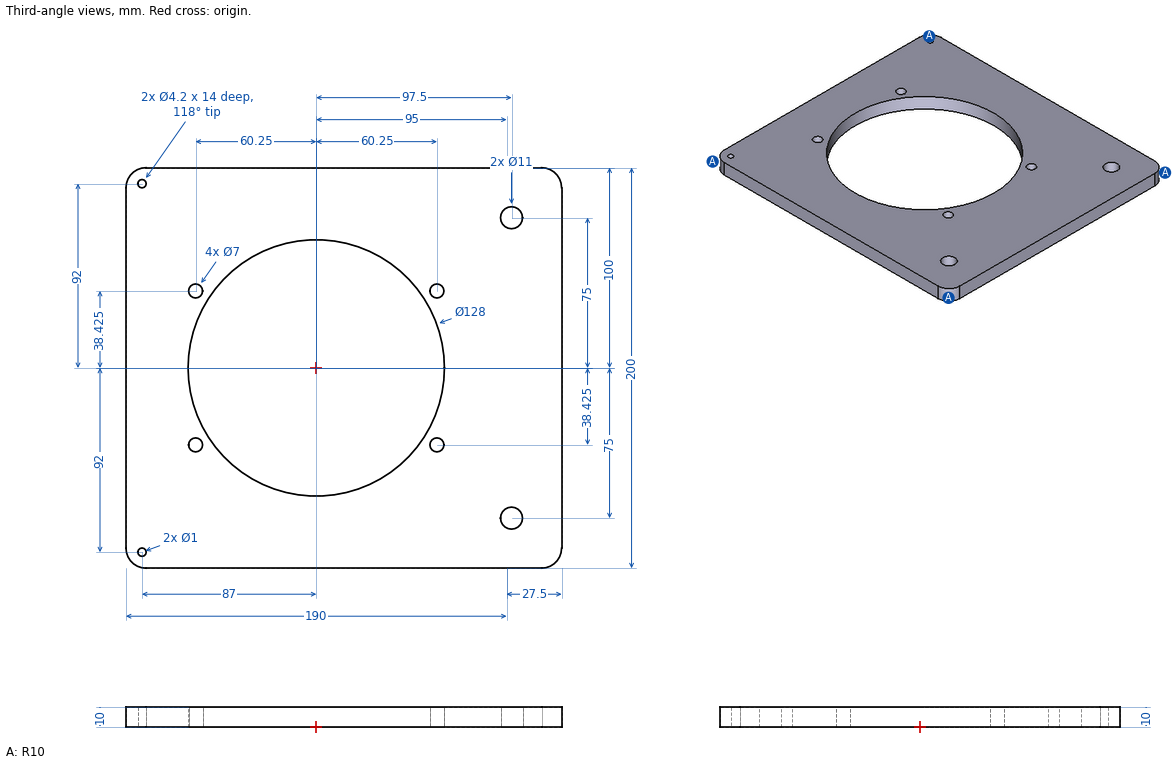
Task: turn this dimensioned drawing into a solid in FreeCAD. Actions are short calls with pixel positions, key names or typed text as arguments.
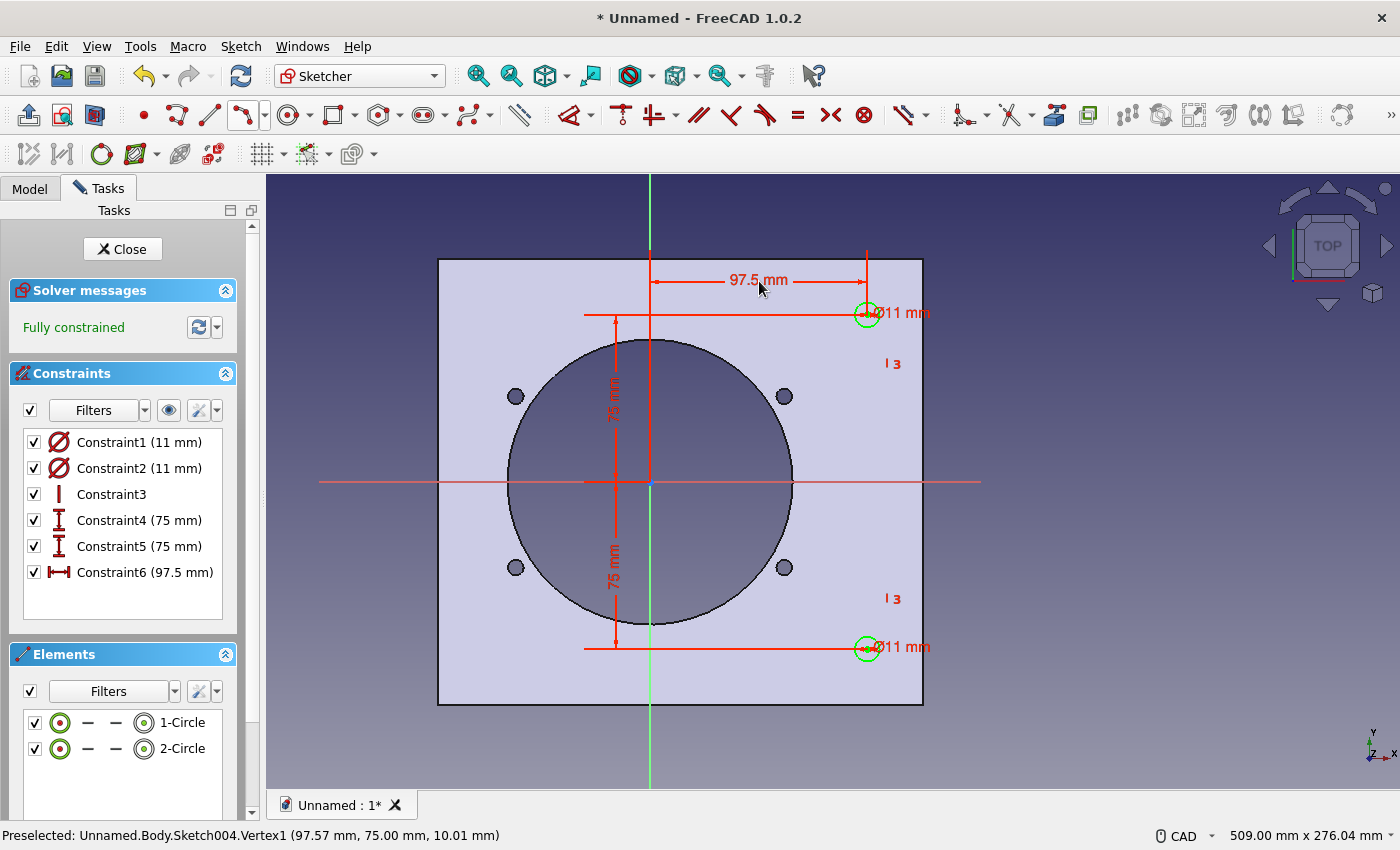
click(123, 249)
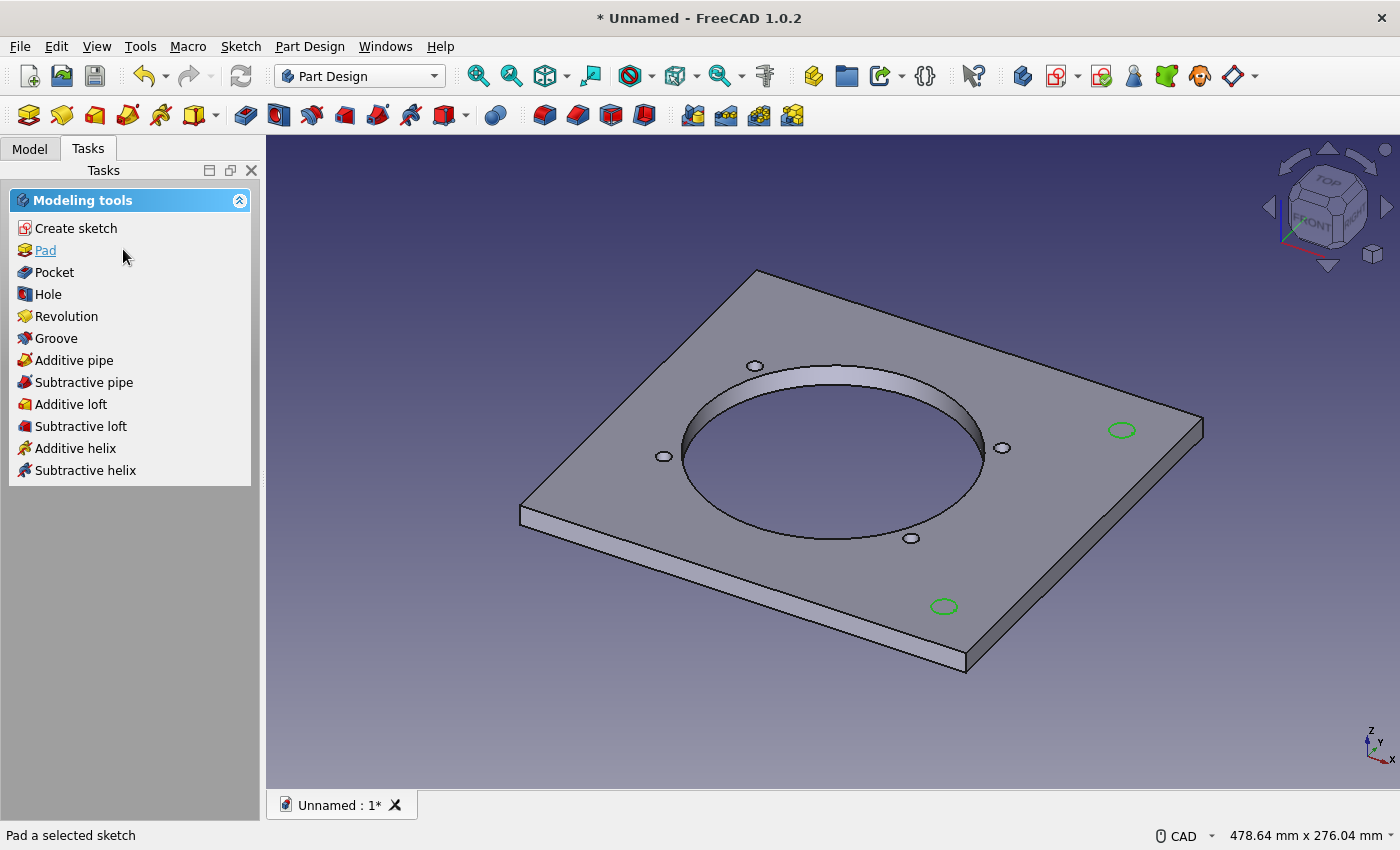
click(246, 116)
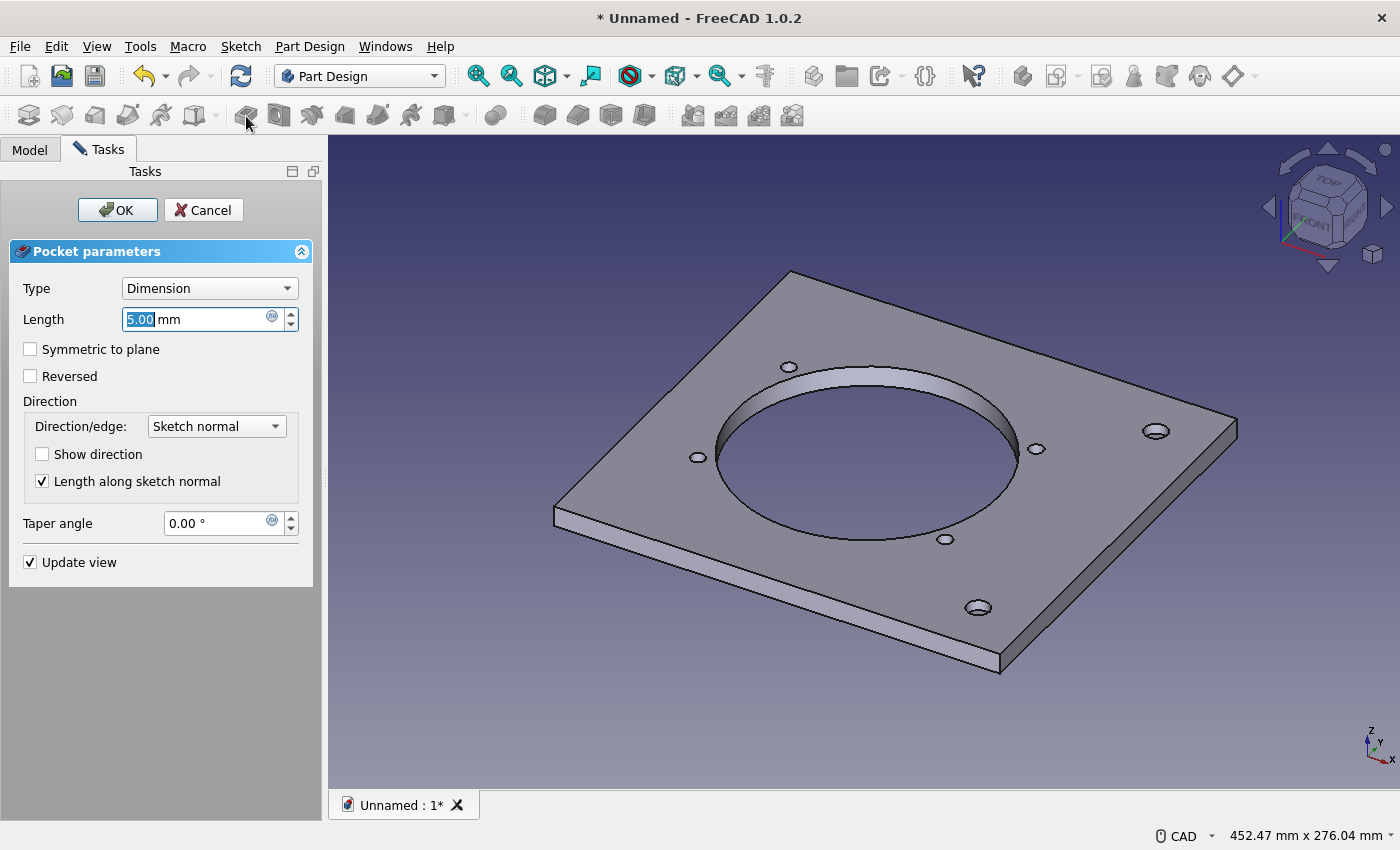
text(10)
key(Tab)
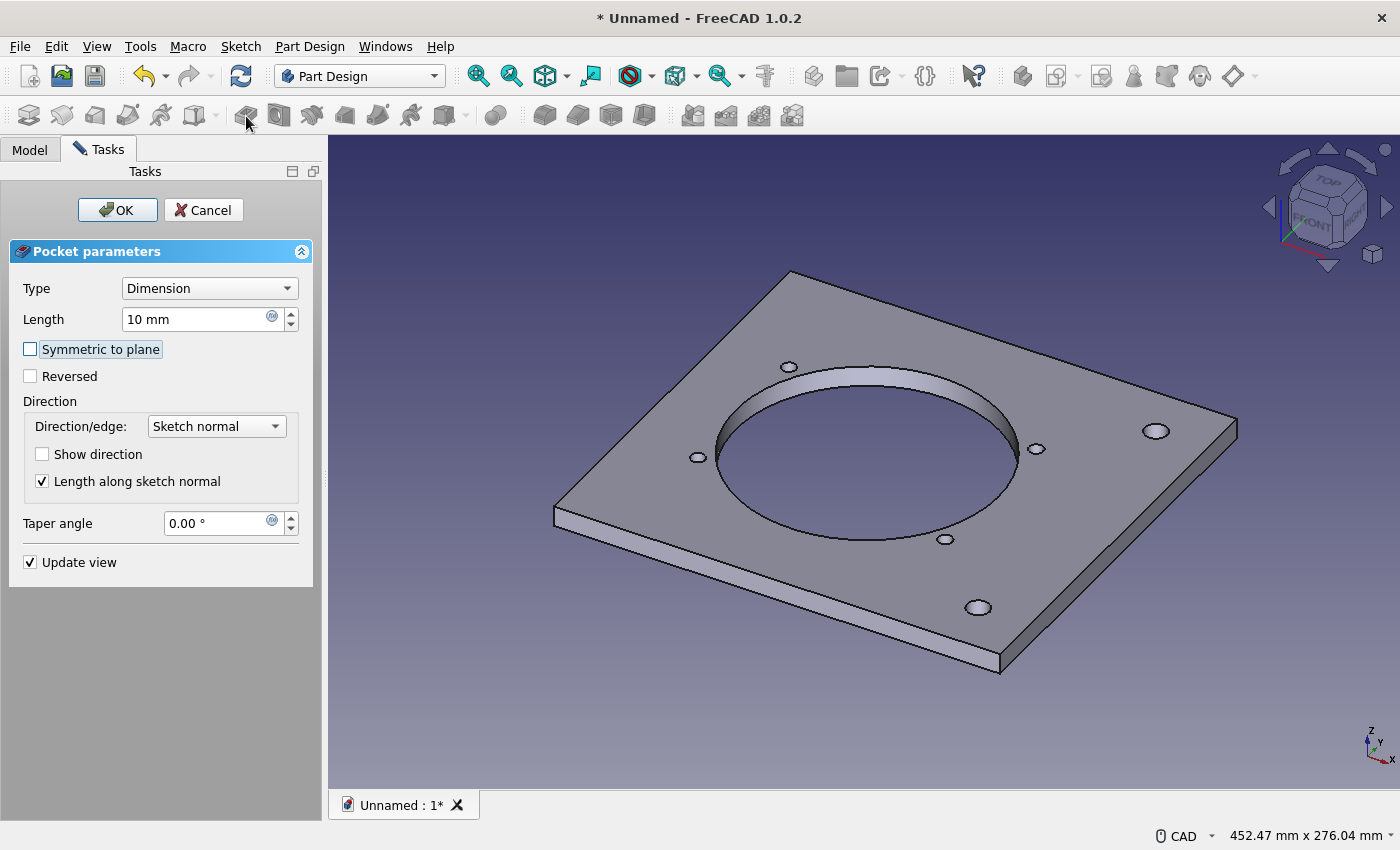
click(118, 210)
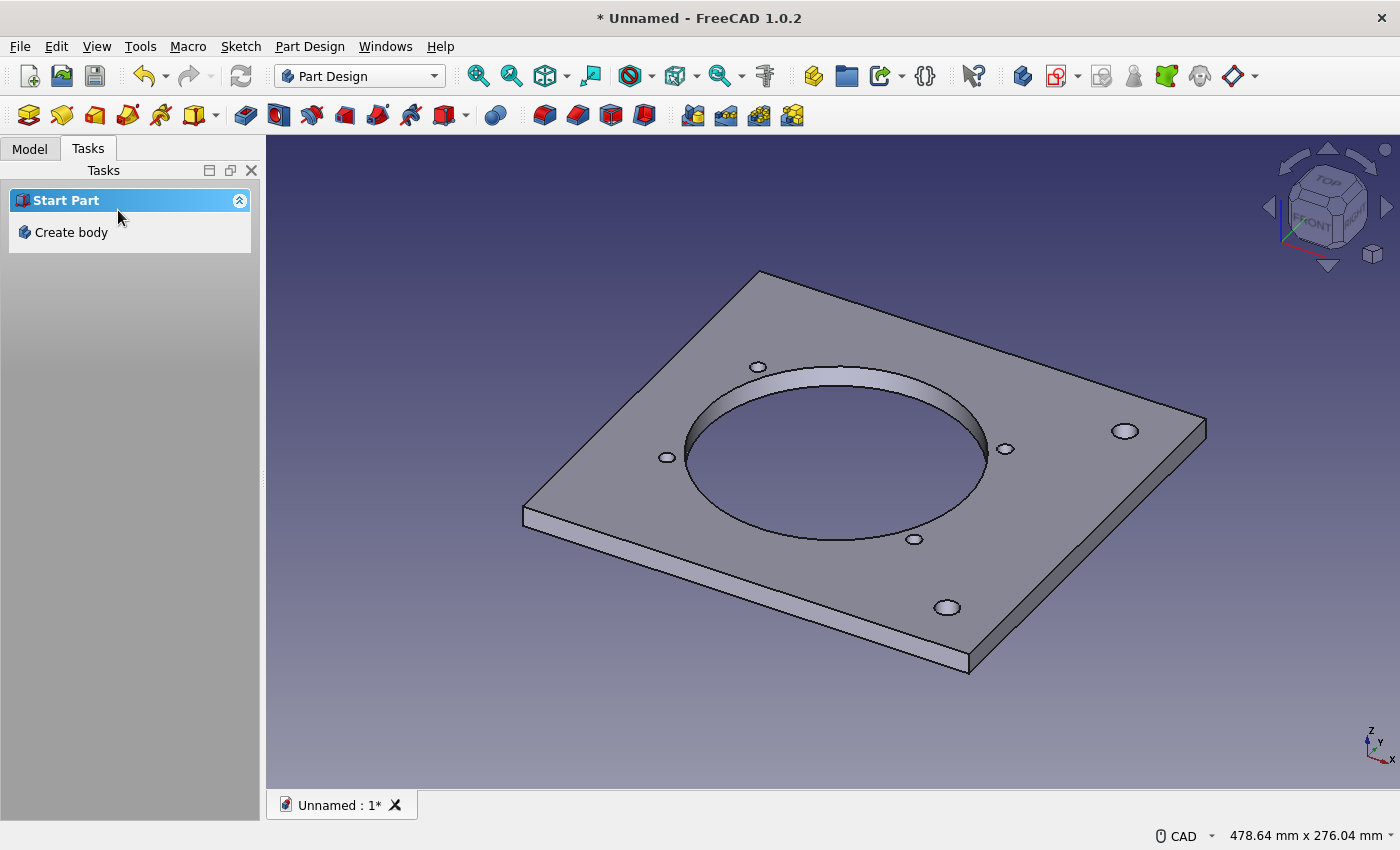
click(924, 571)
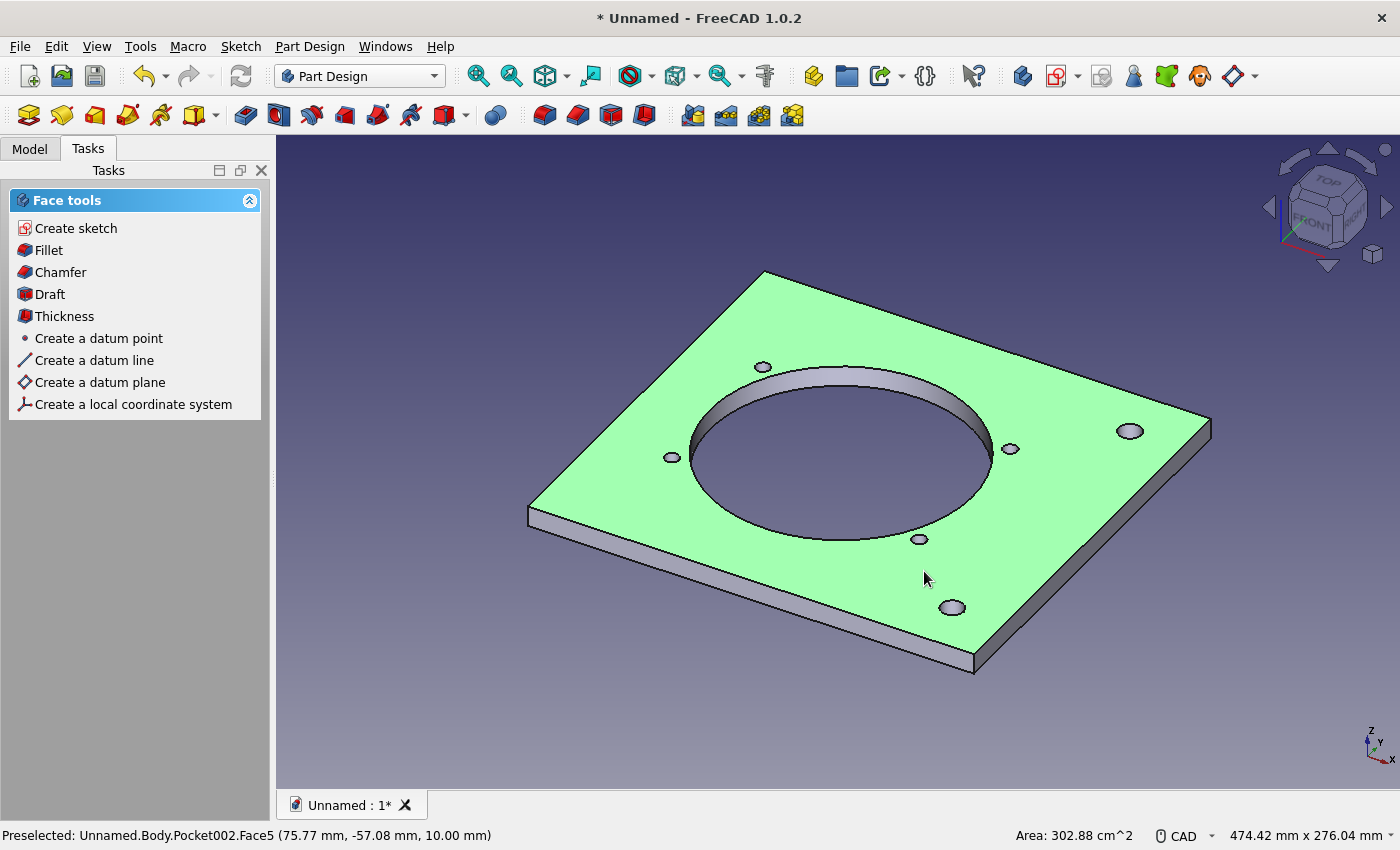
click(1056, 76)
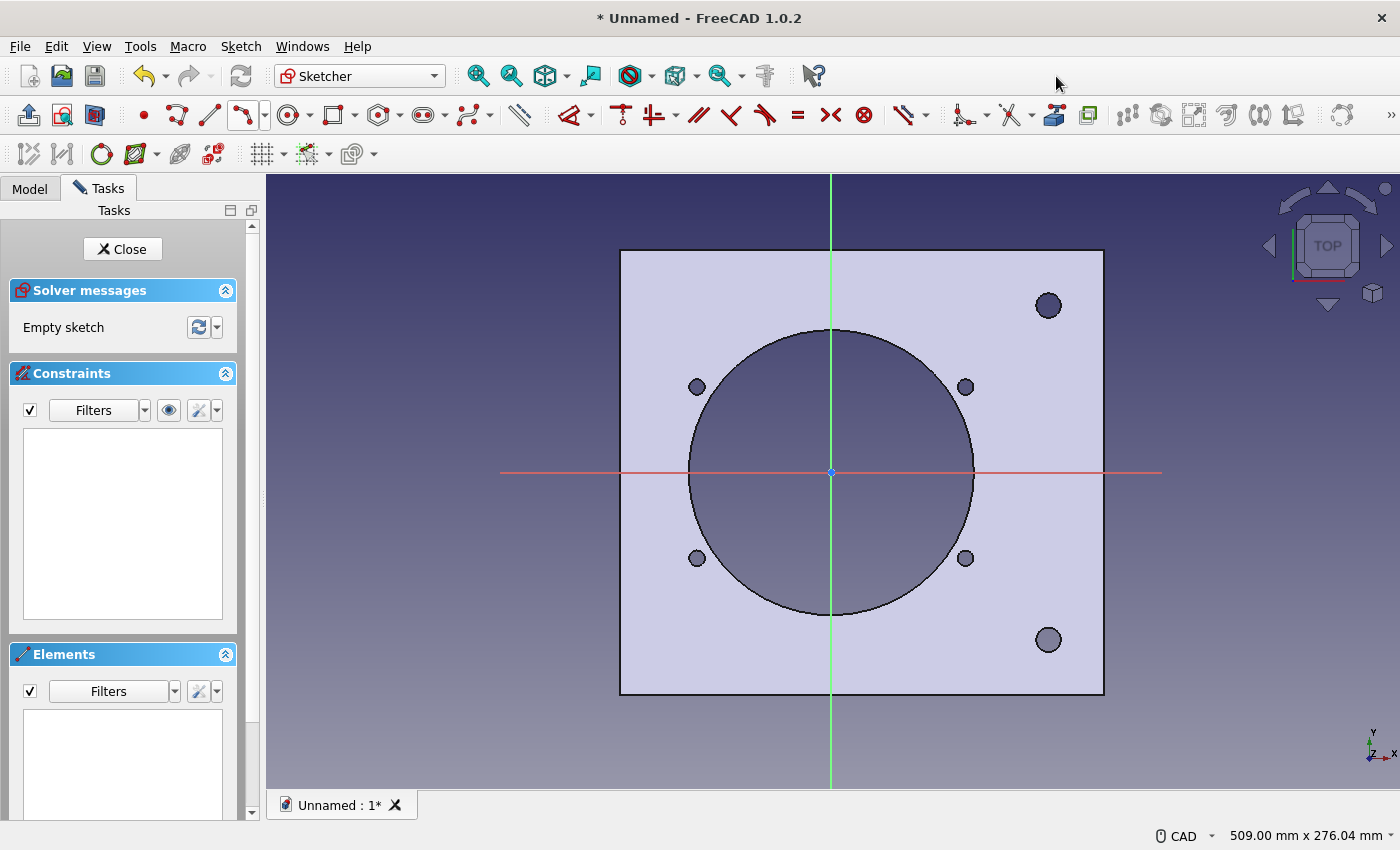
click(288, 116)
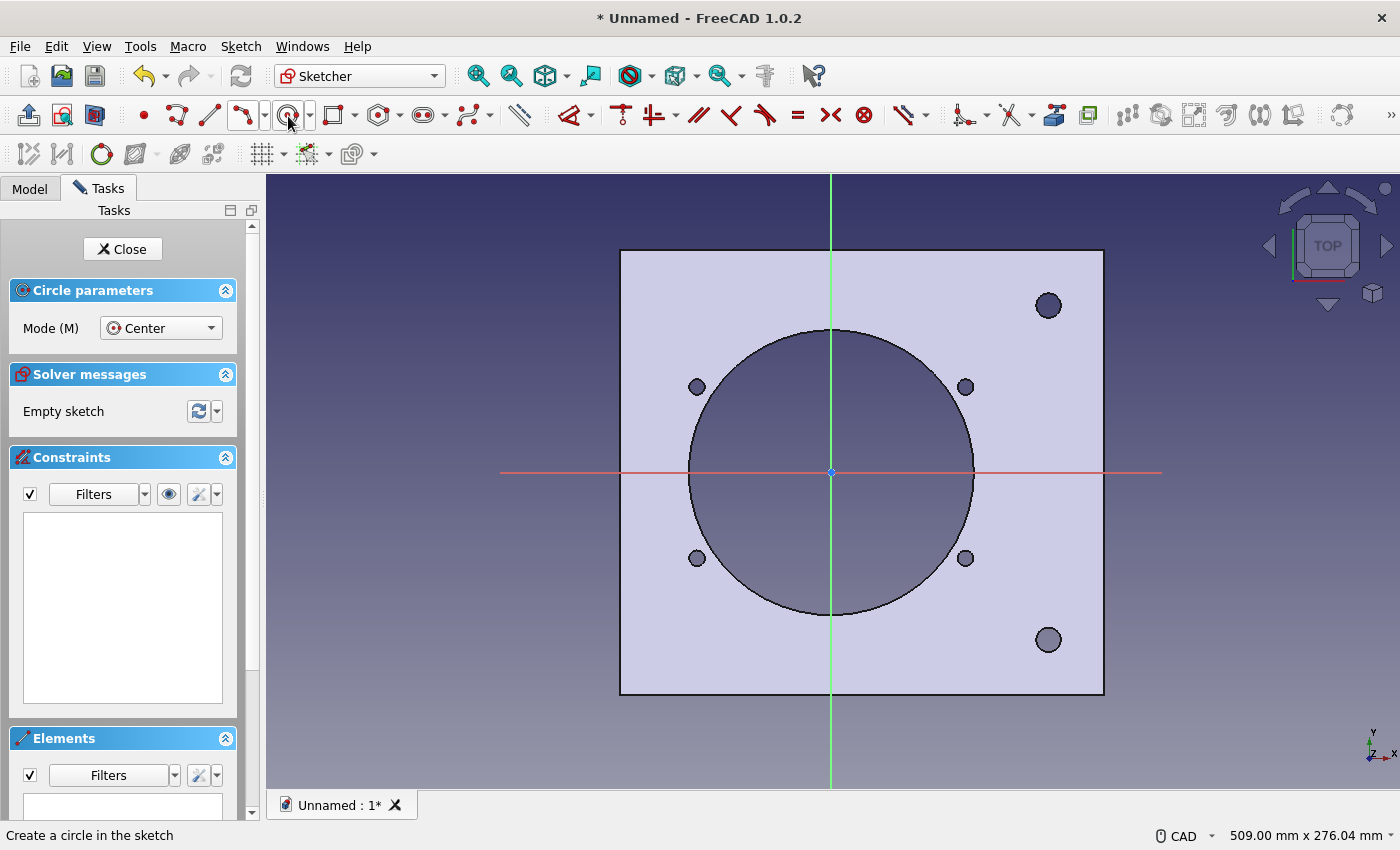
scroll(637, 678, up, 16)